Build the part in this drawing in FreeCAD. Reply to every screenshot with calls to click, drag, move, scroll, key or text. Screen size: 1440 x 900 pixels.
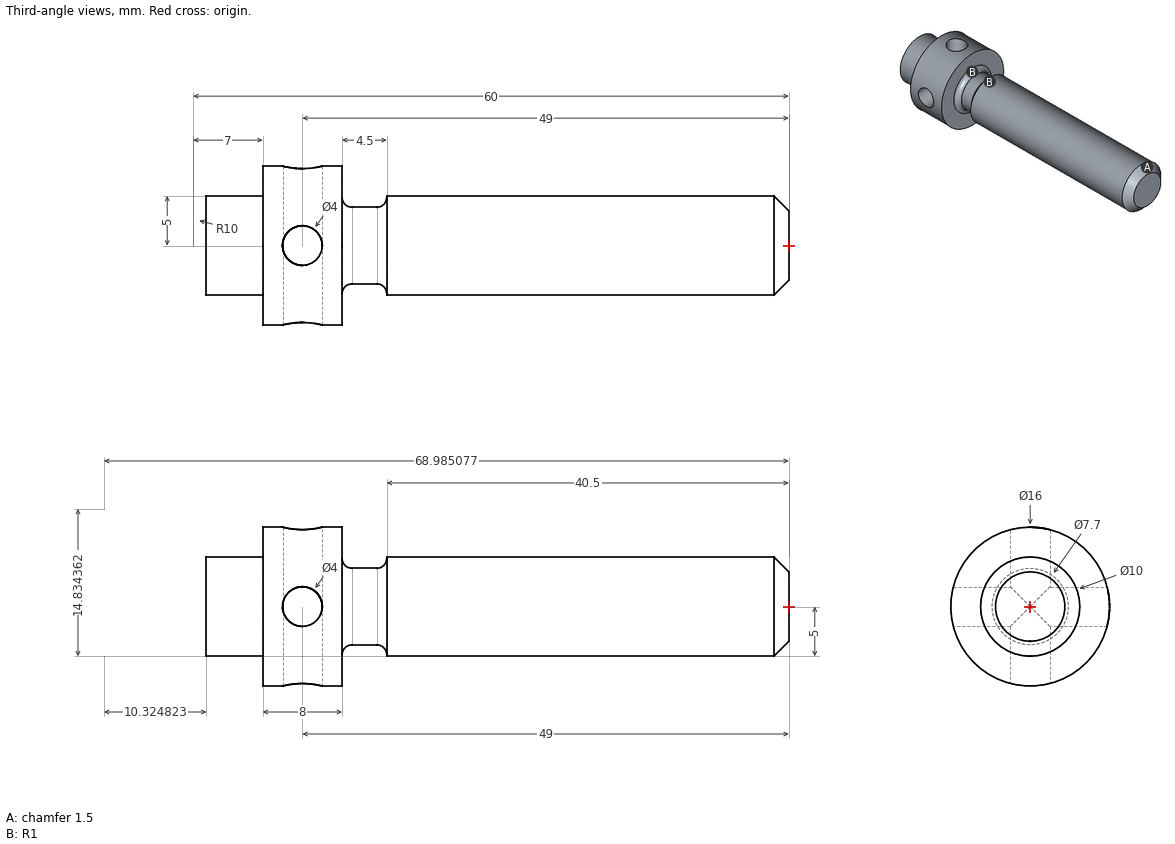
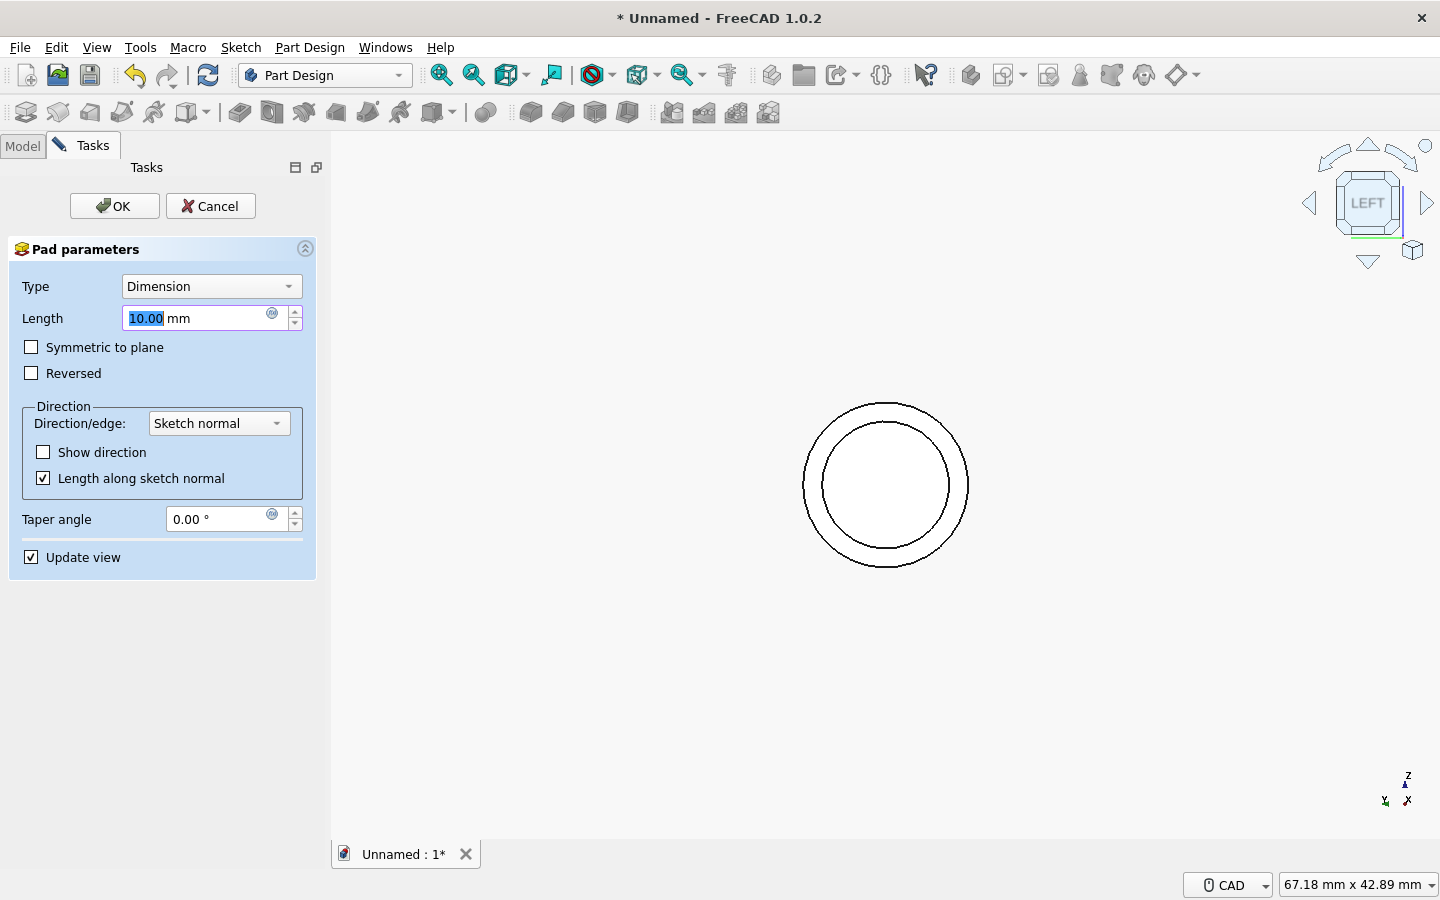
text(4.5)
key(Tab)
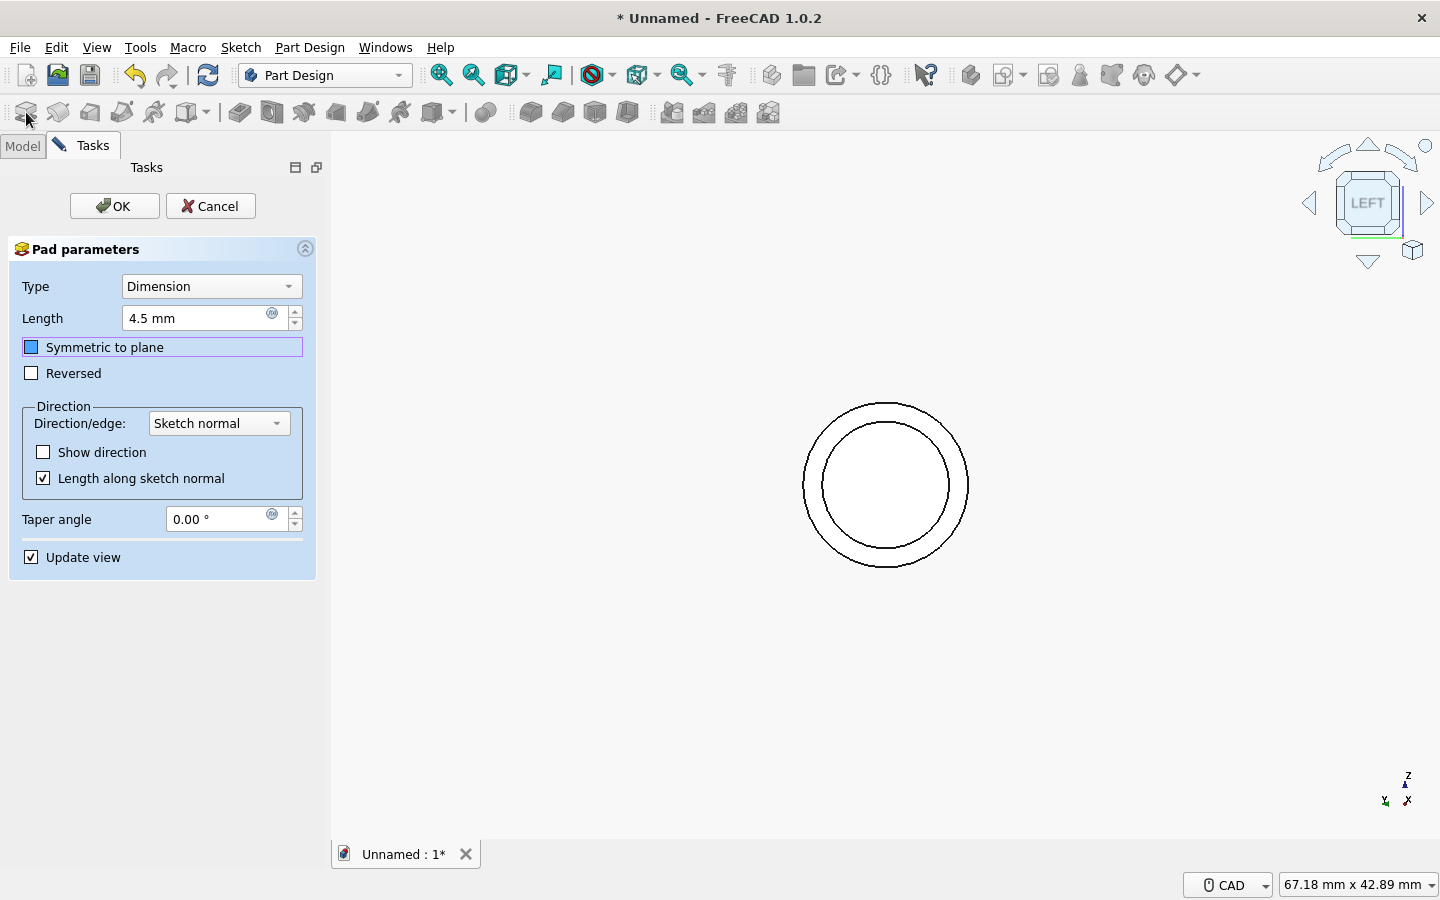
click(115, 206)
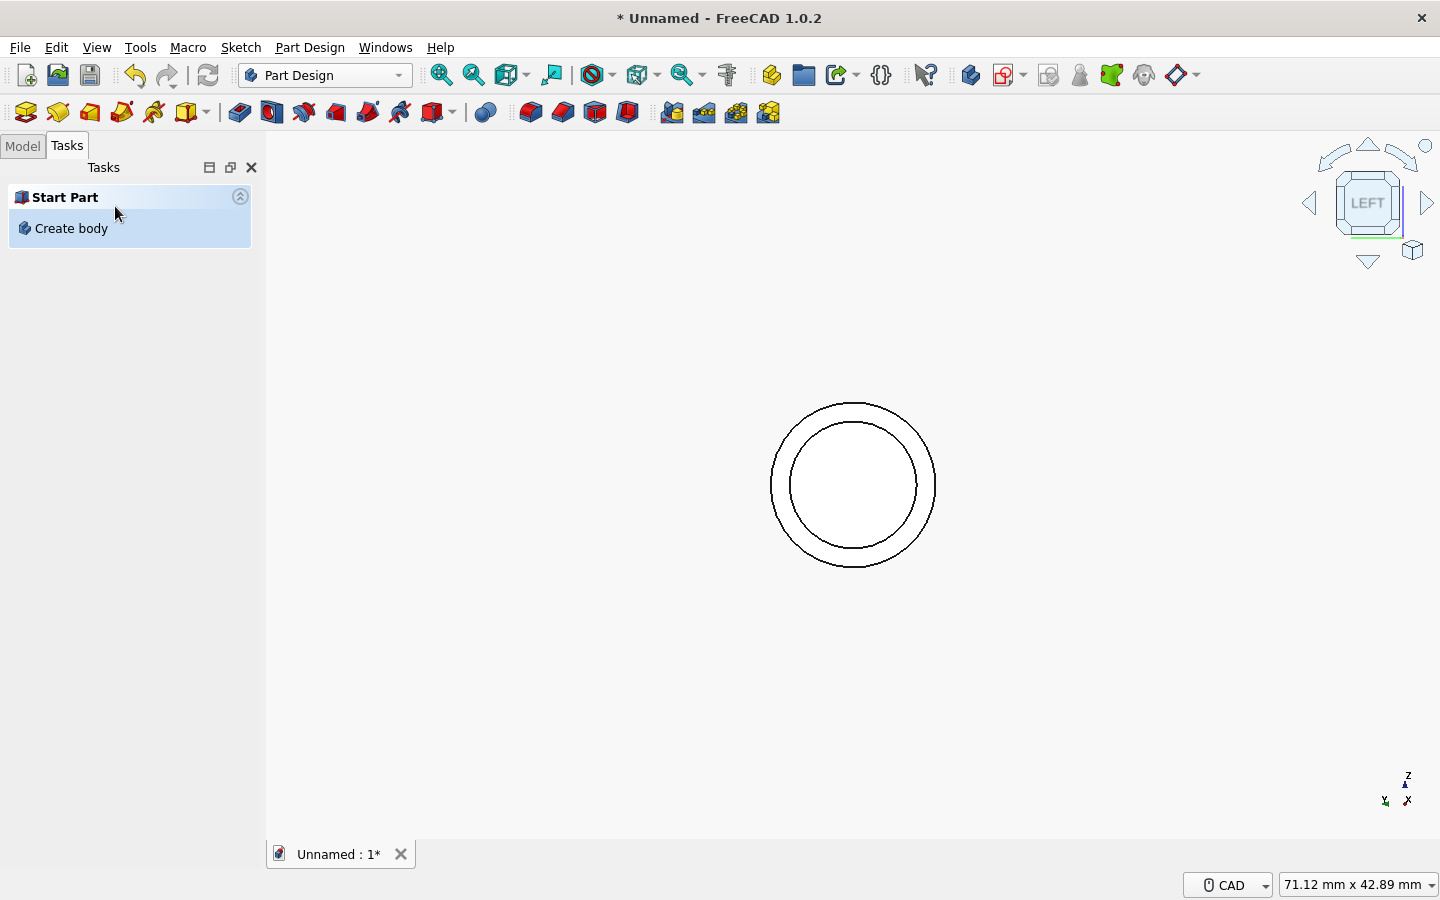
key(v)
key(f)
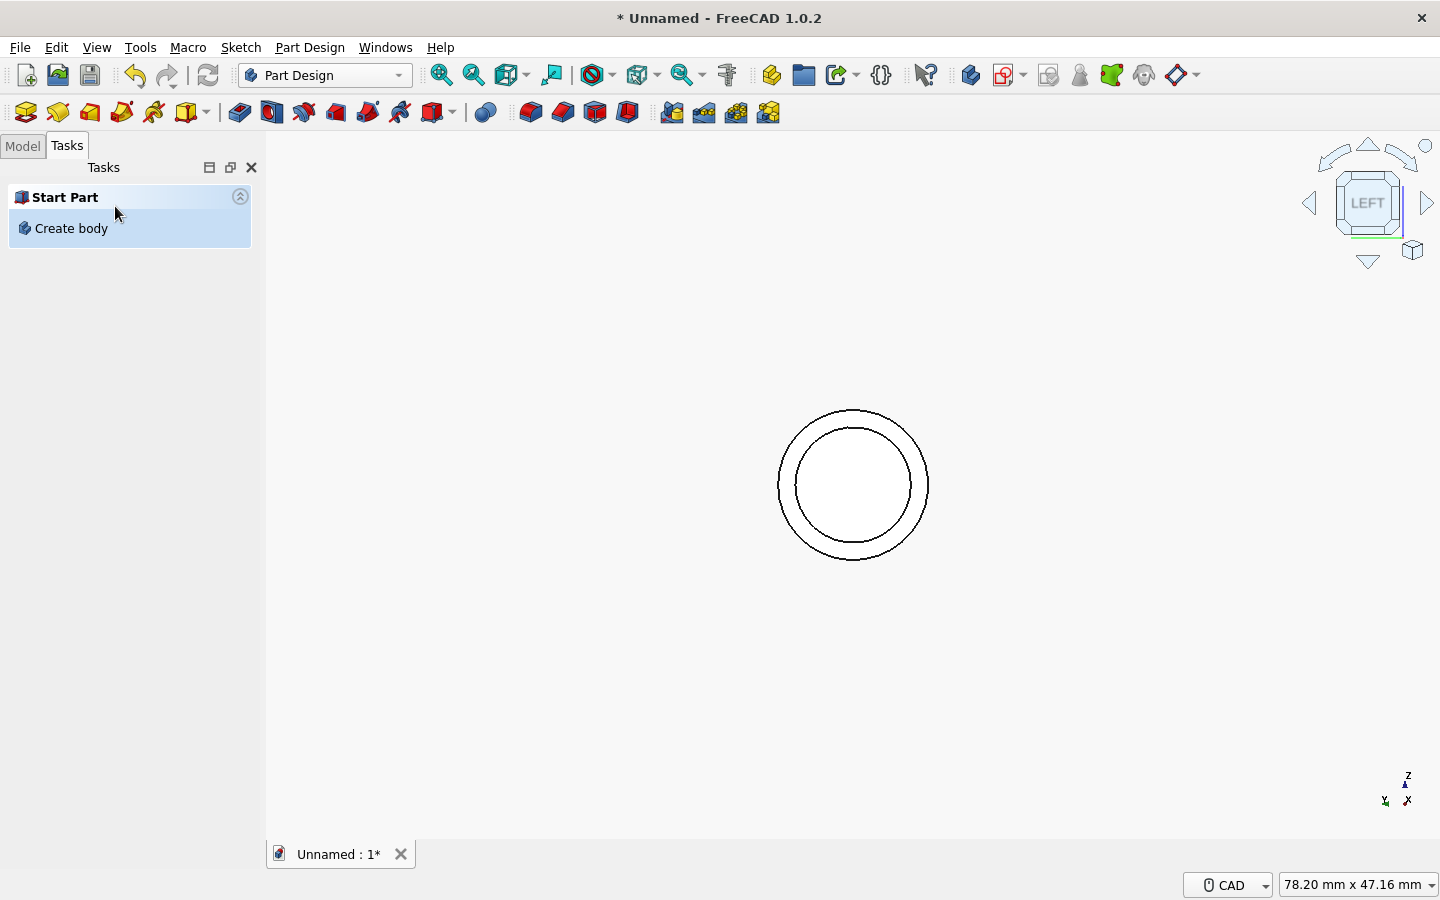
click(853, 484)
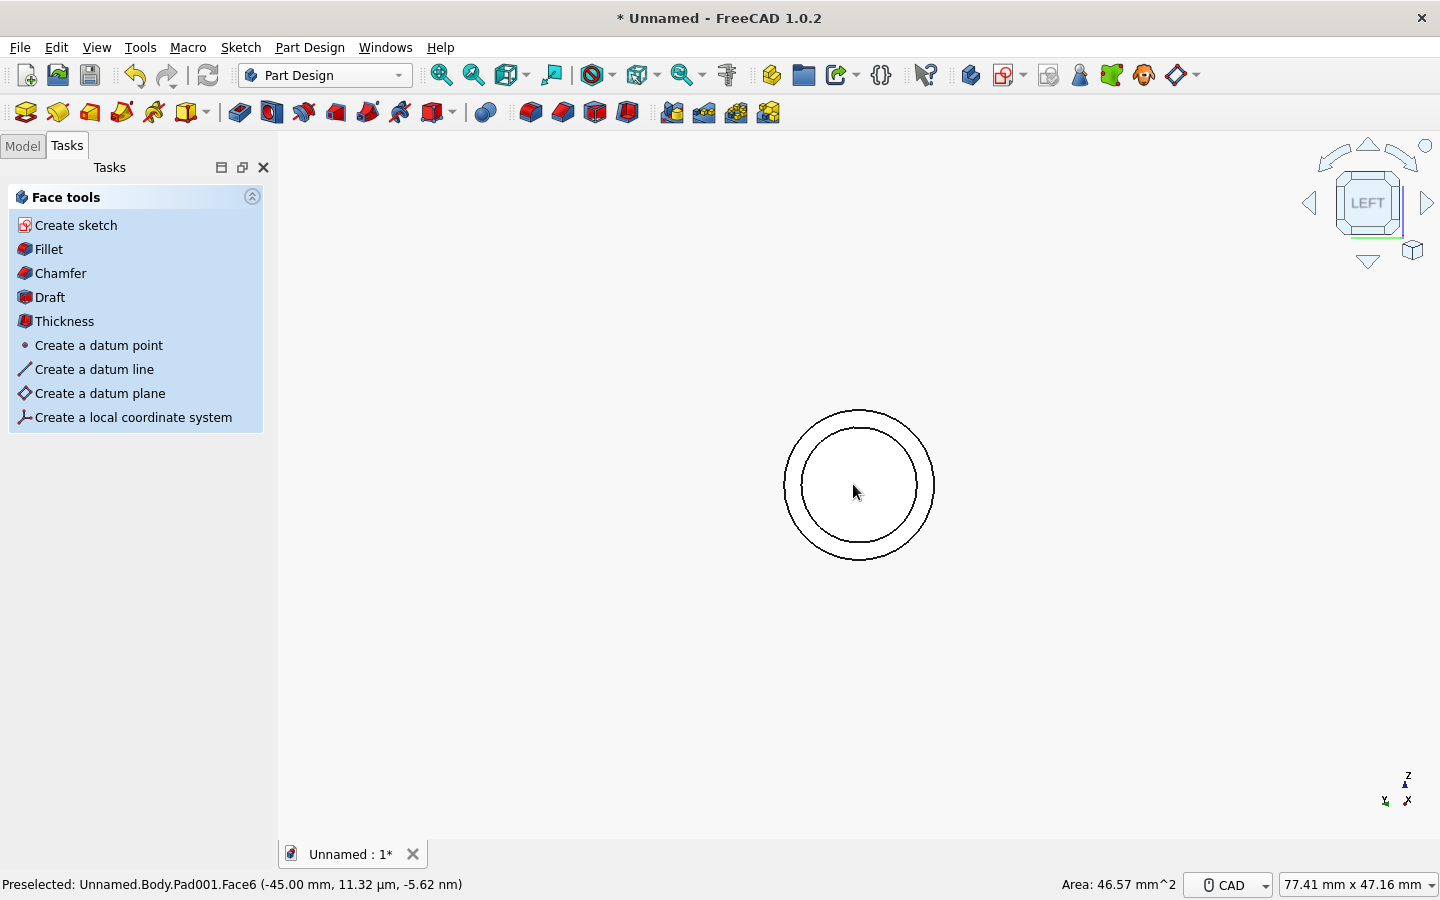
click(1004, 76)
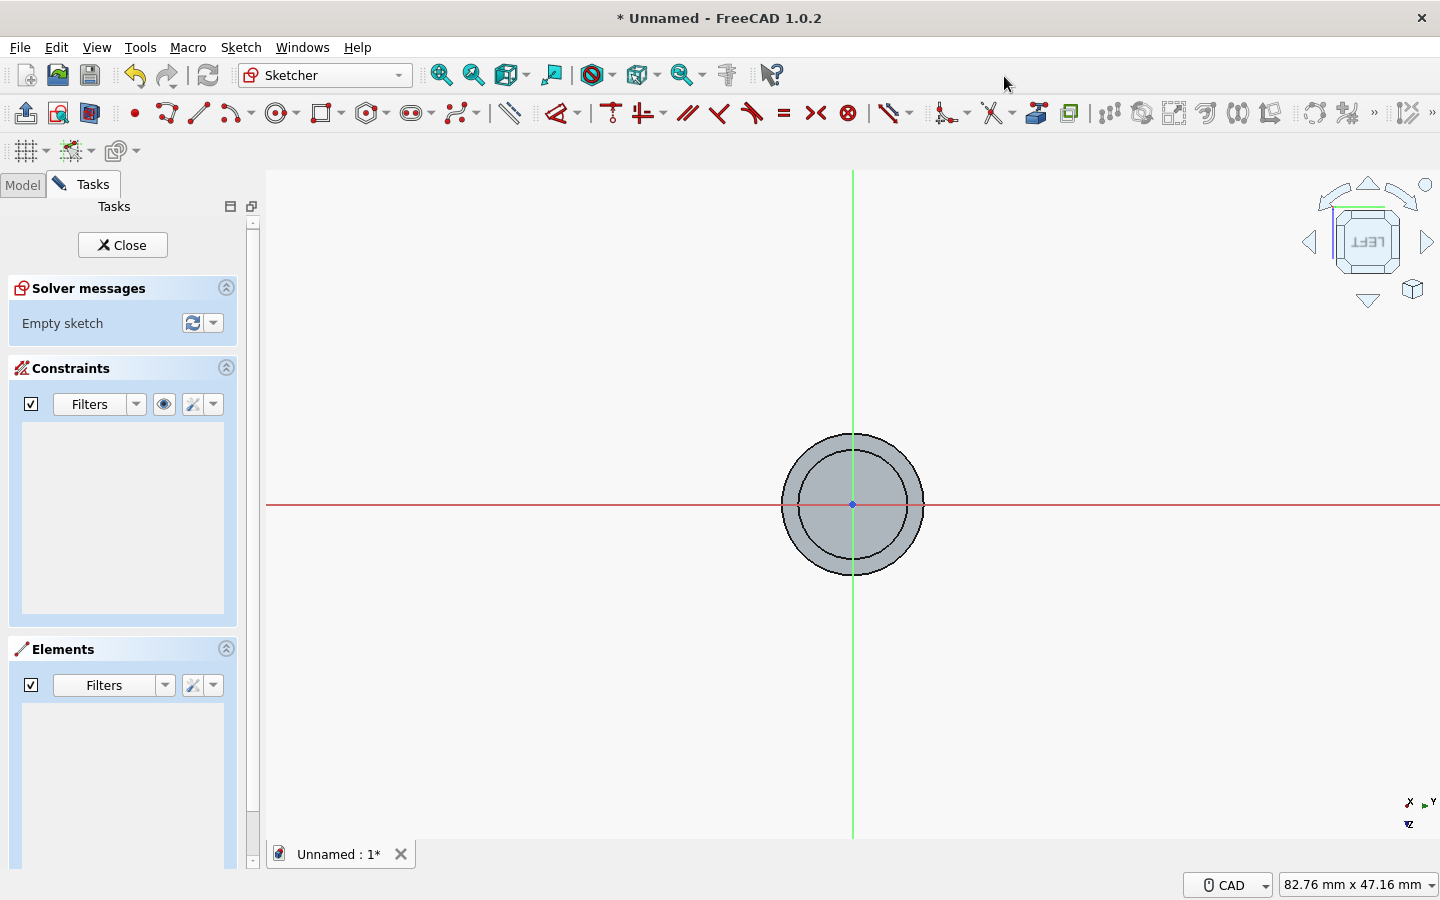
scroll(936, 505, up, 3)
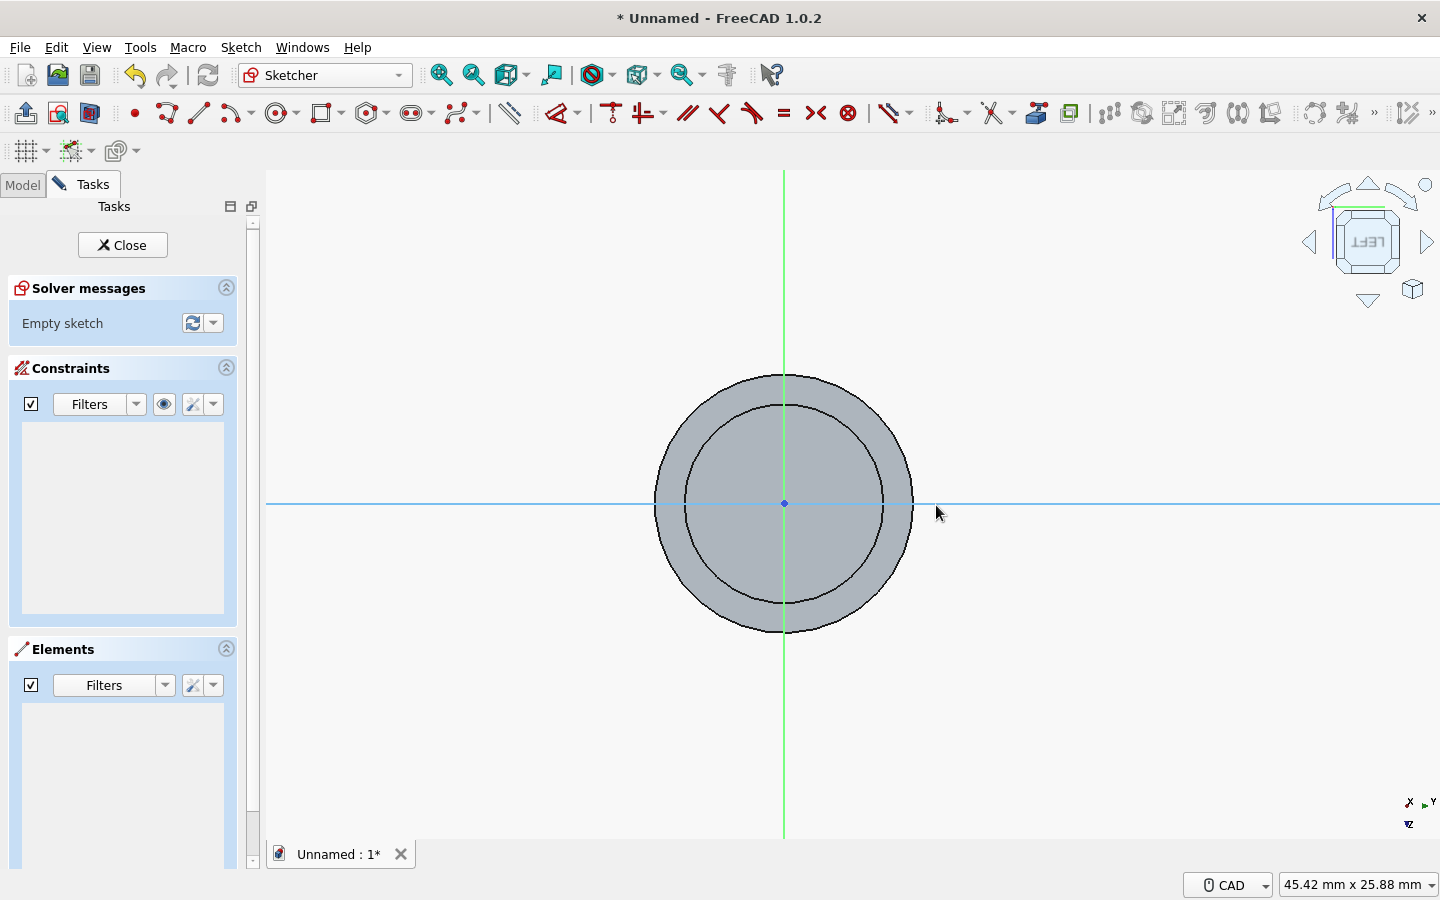
click(276, 114)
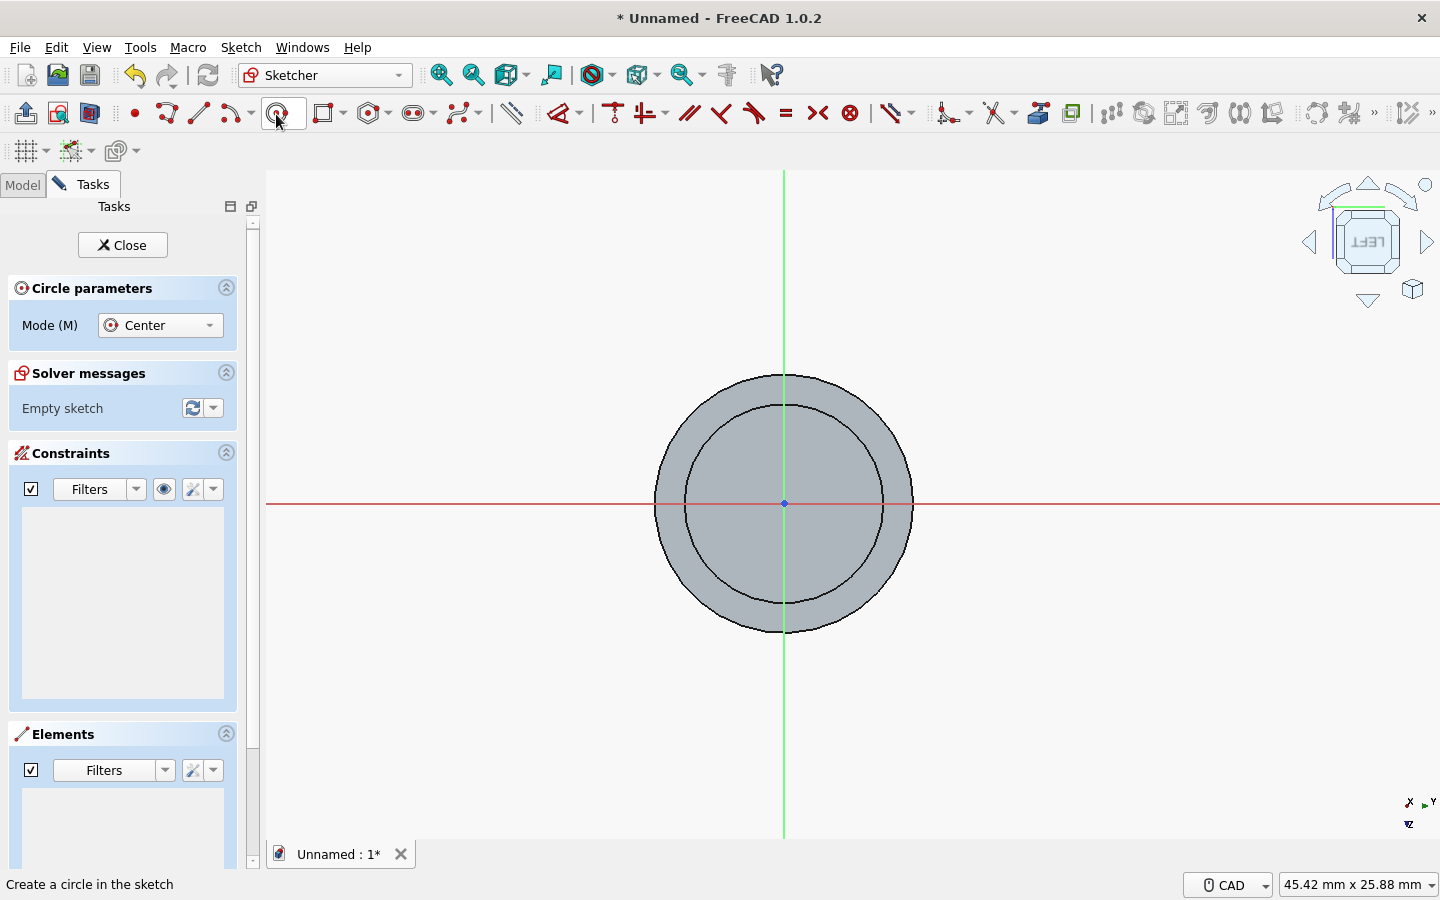
click(784, 504)
click(930, 357)
key(Escape)